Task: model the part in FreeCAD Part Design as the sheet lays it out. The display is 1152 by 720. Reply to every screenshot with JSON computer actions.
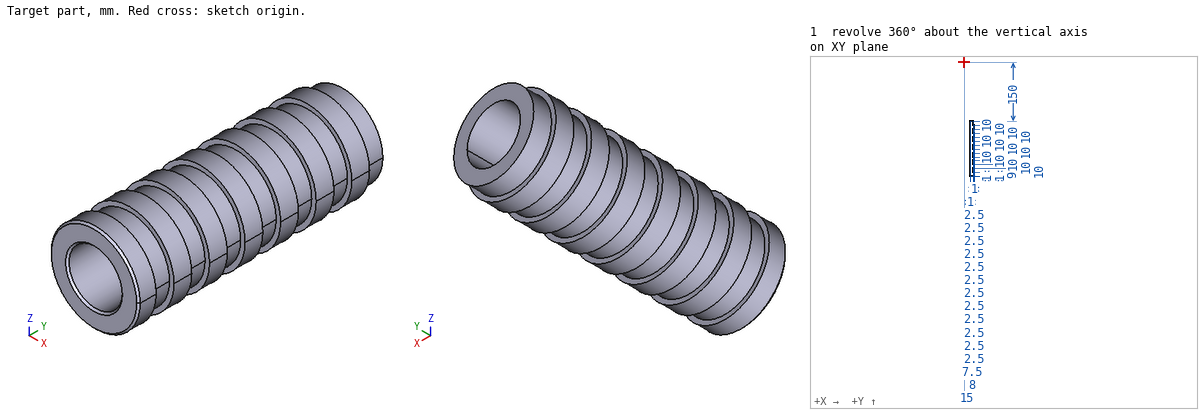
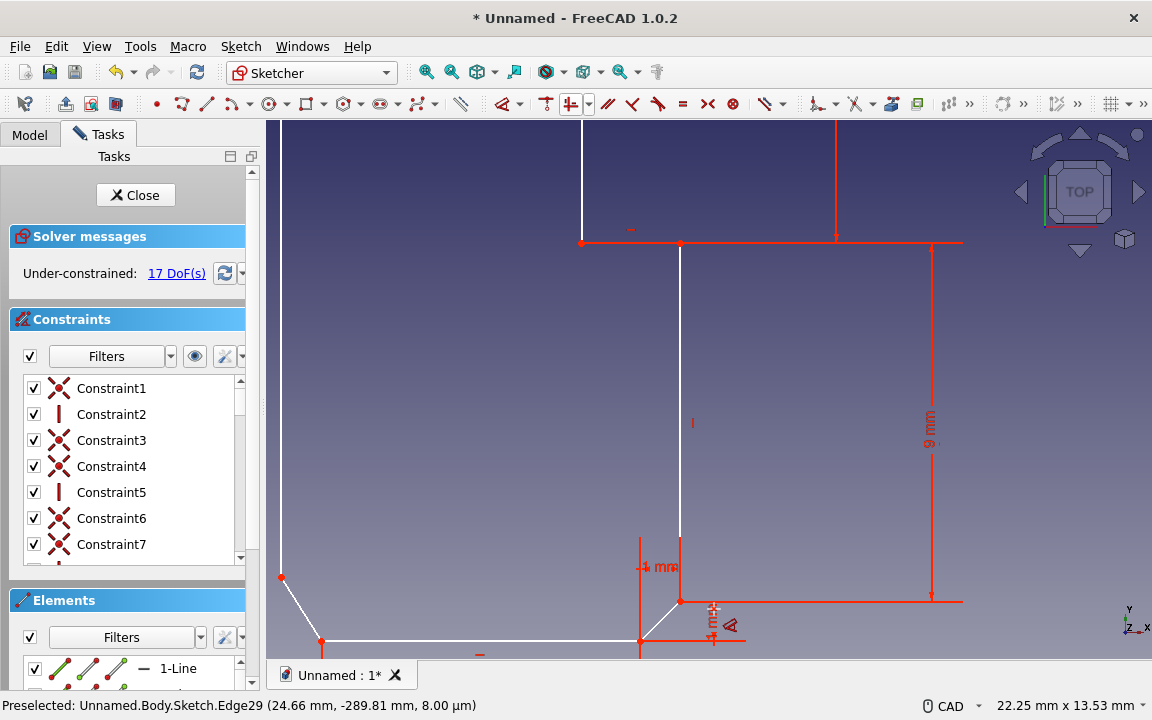
{"action": "left_click", "coordinate": [310, 622]}
{"action": "left_click", "coordinate": [308, 544]}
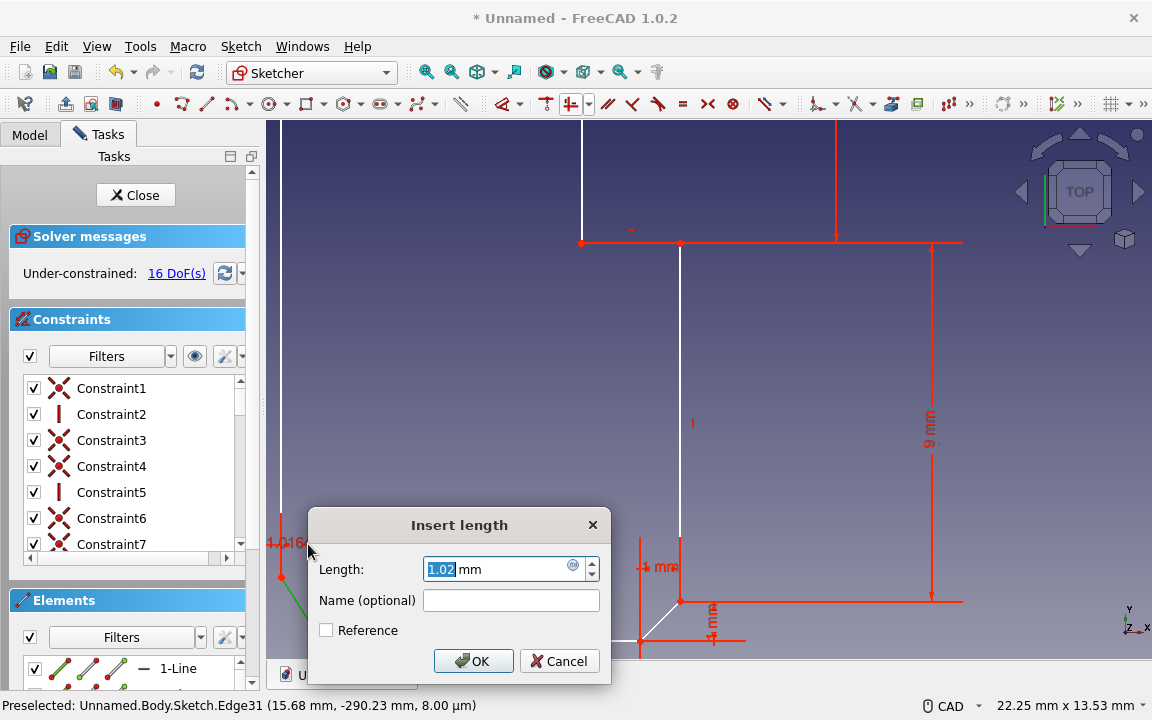
{"action": "type", "text": "1"}
{"action": "key", "text": "Return"}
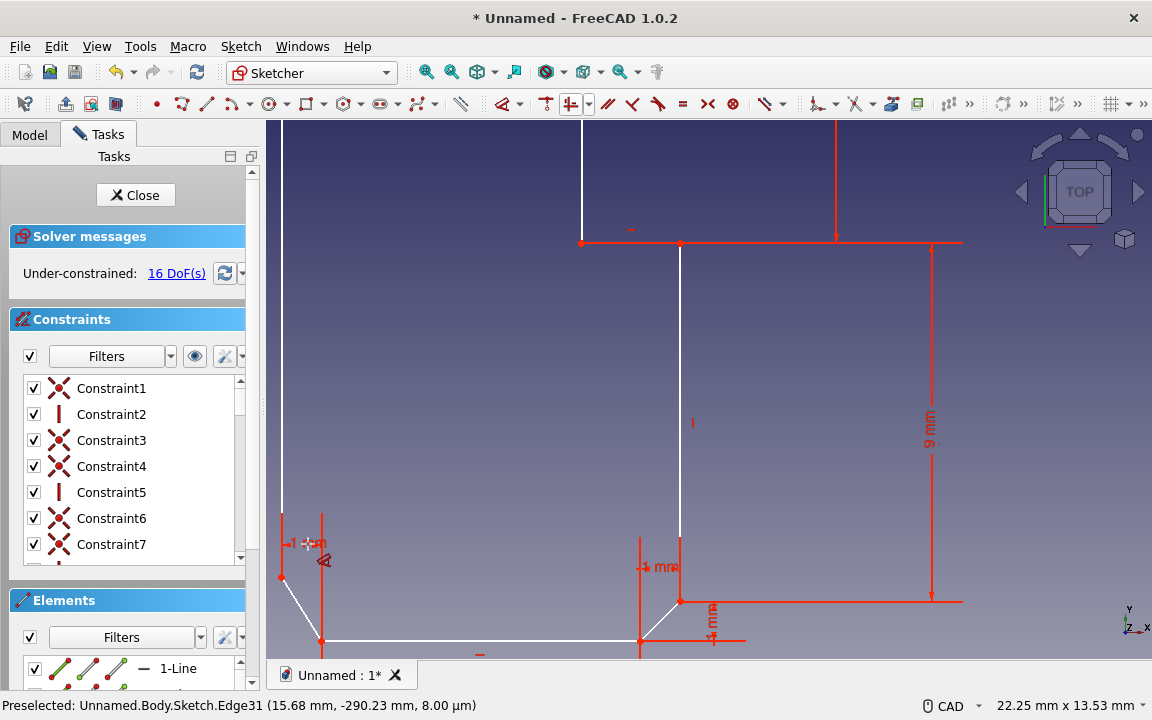
{"action": "left_click", "coordinate": [310, 622]}
{"action": "left_click", "coordinate": [356, 604]}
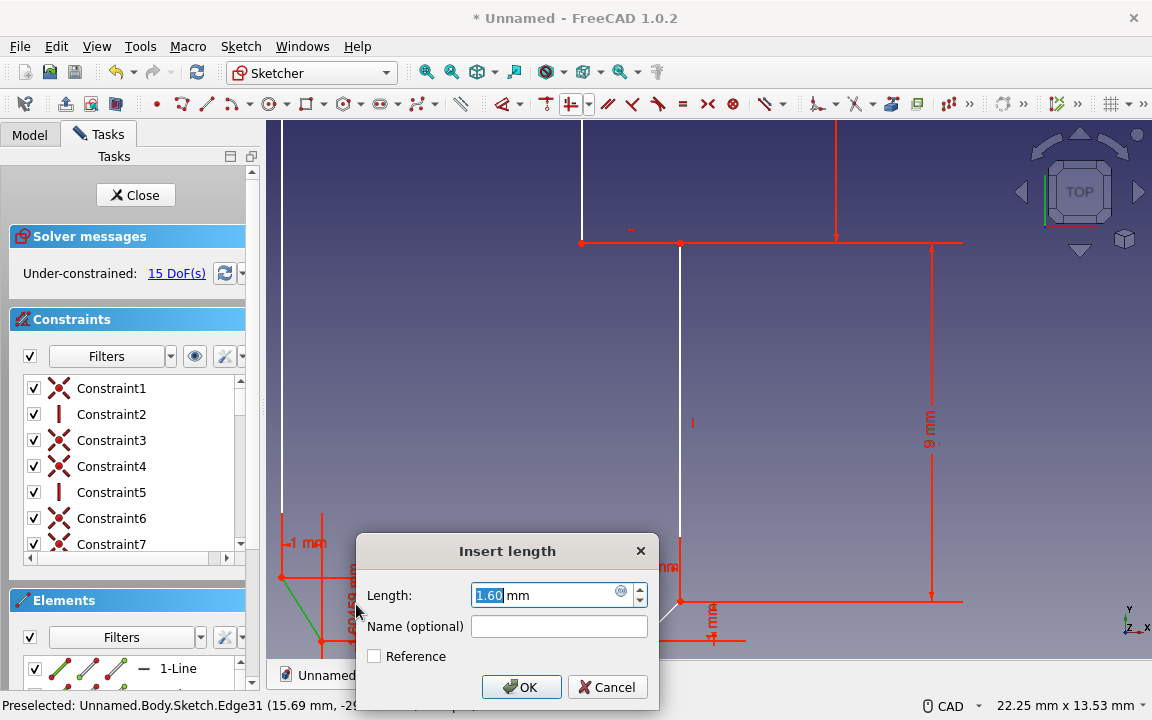
{"action": "type", "text": "1"}
{"action": "key", "text": "Return"}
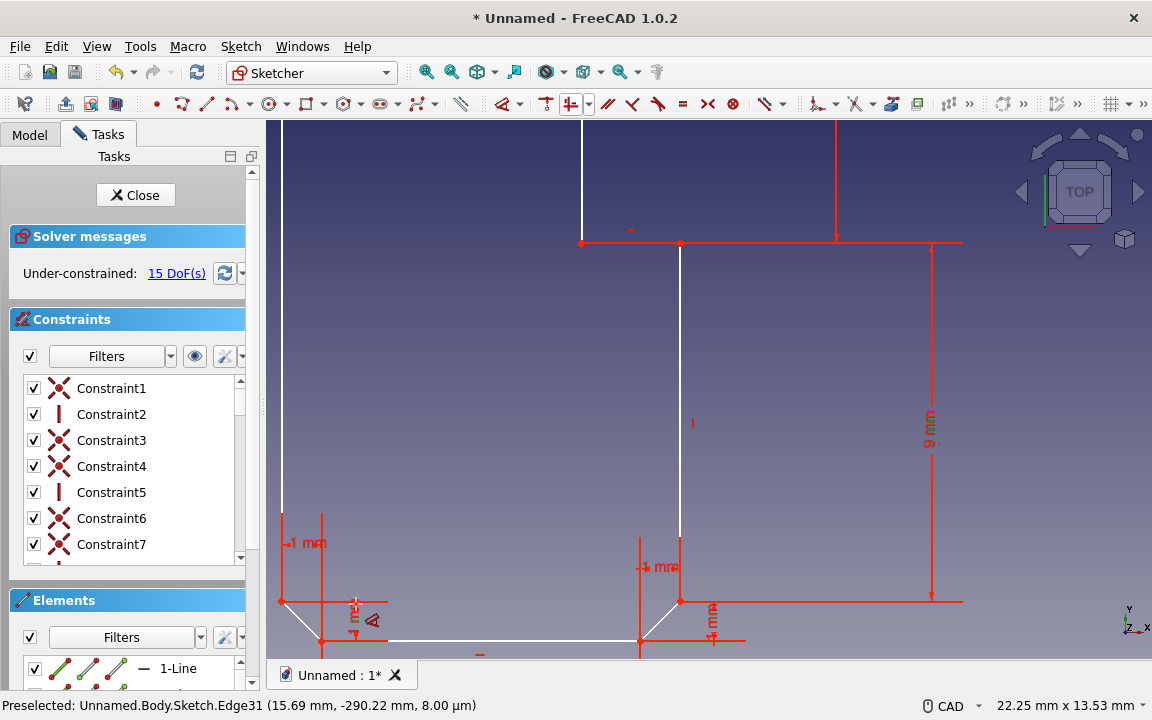
{"action": "scroll", "coordinate": [656, 581], "scroll_direction": "down", "scroll_amount": 17}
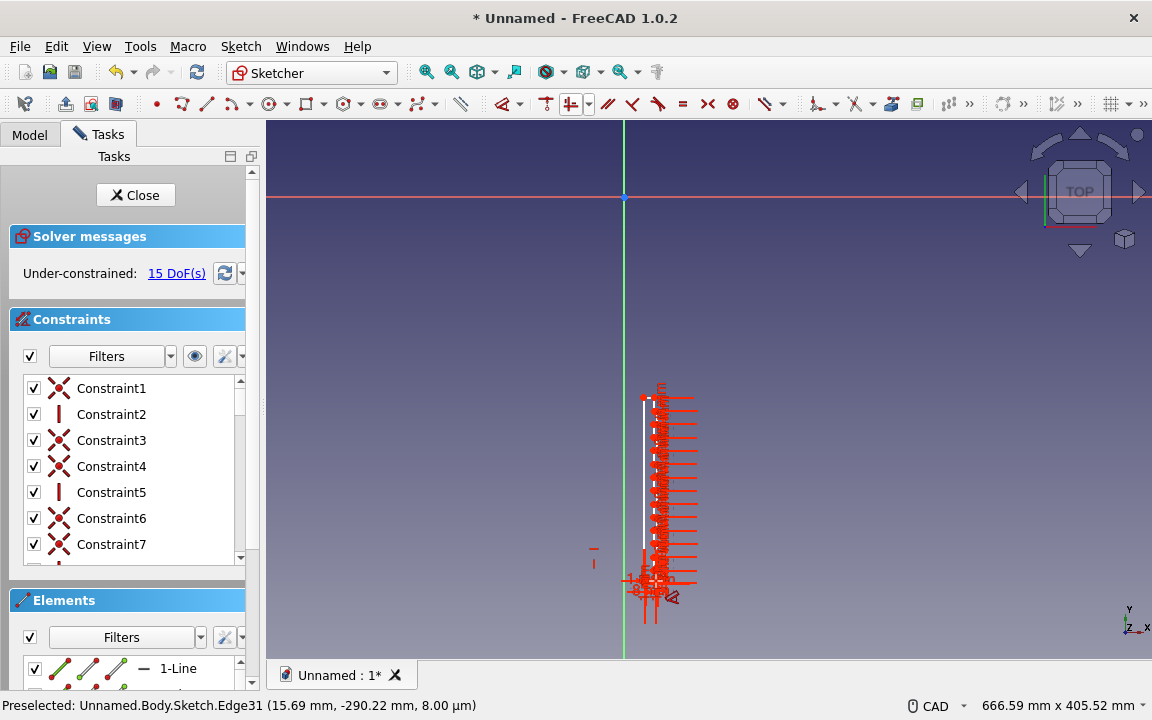
{"action": "scroll", "coordinate": [647, 398], "scroll_direction": "up", "scroll_amount": 8}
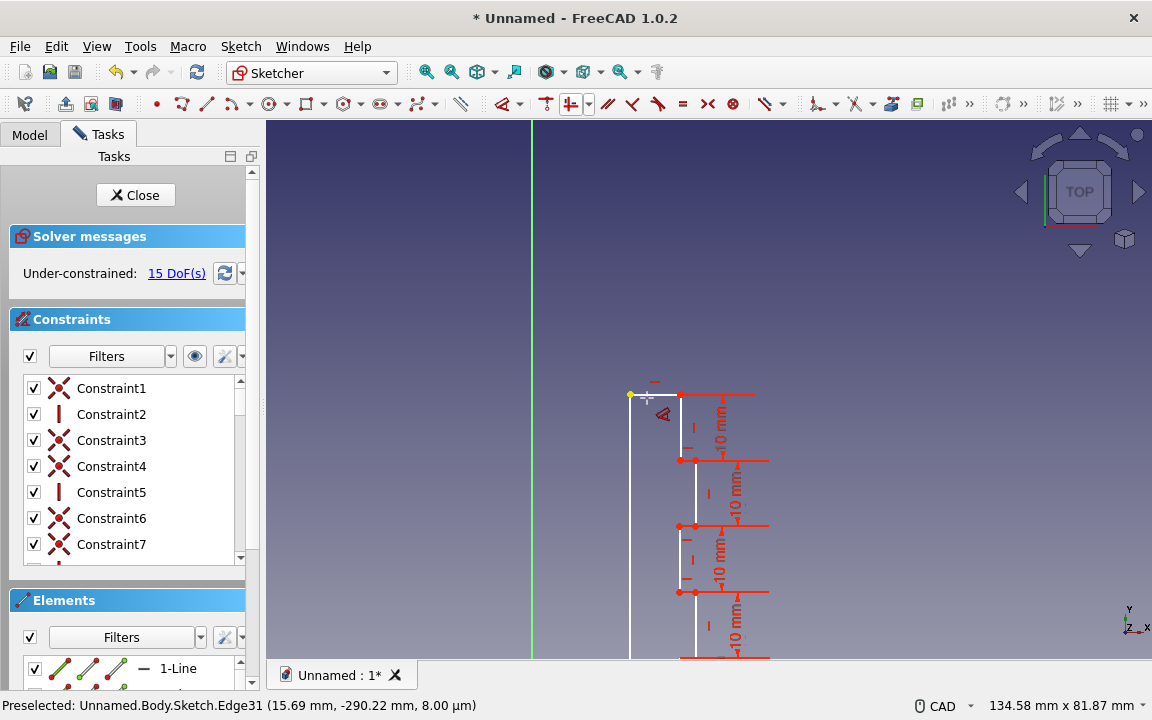
{"action": "left_click", "coordinate": [645, 395]}
{"action": "left_click", "coordinate": [644, 429]}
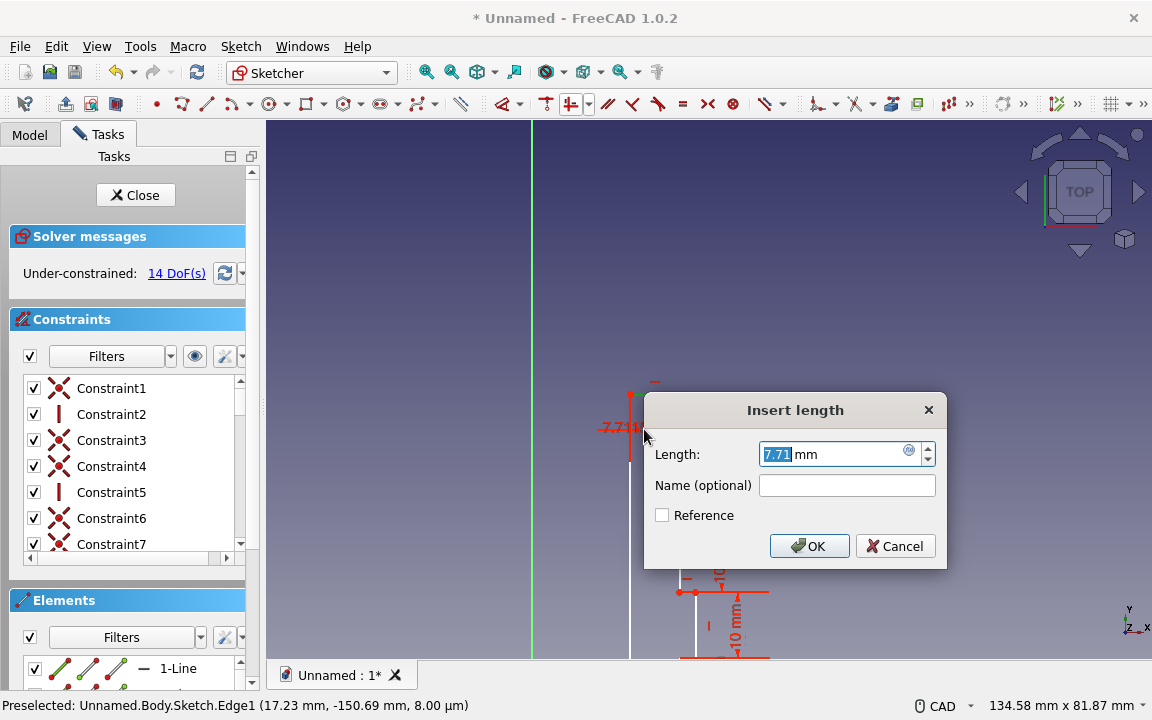
{"action": "type", "text": "7.5"}
{"action": "key", "text": "Return"}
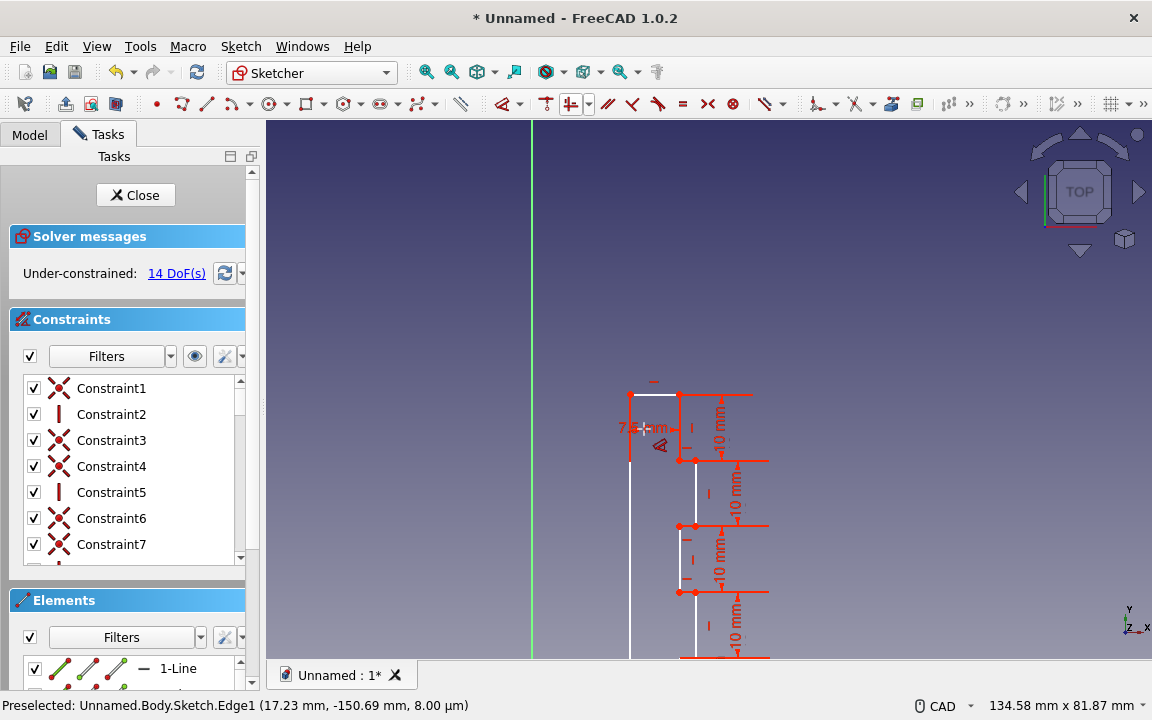
{"action": "scroll", "coordinate": [688, 461], "scroll_direction": "up", "scroll_amount": 5}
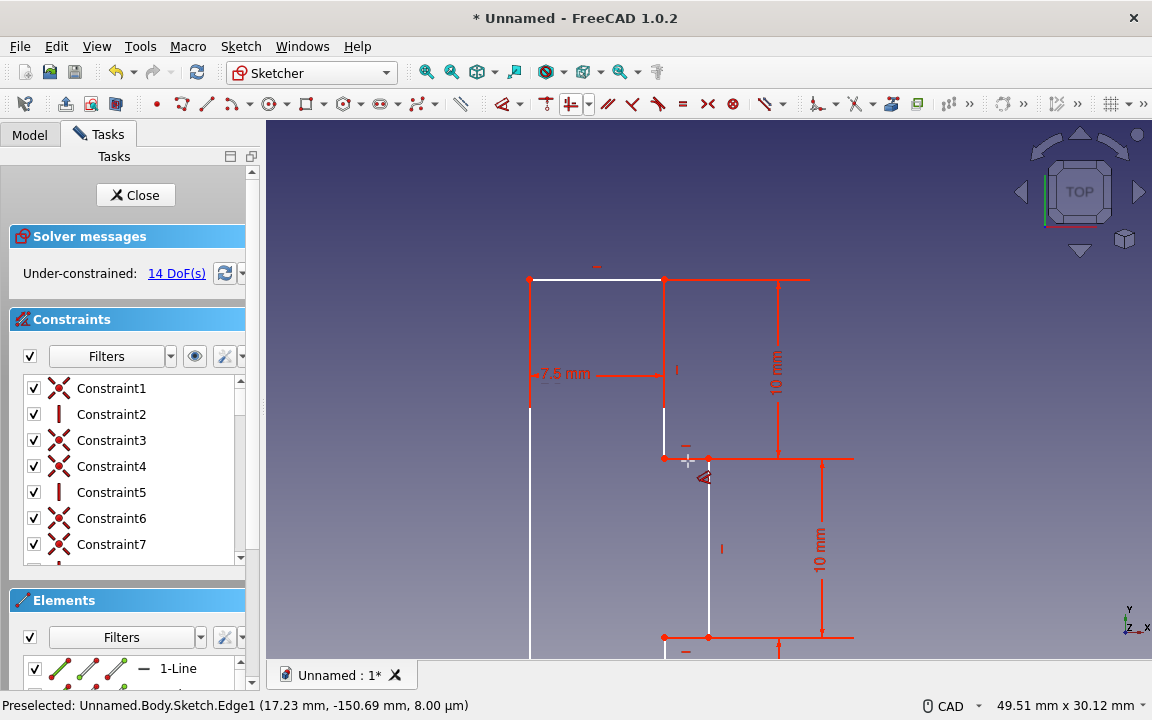
{"action": "left_click", "coordinate": [686, 459]}
{"action": "left_click", "coordinate": [686, 493]}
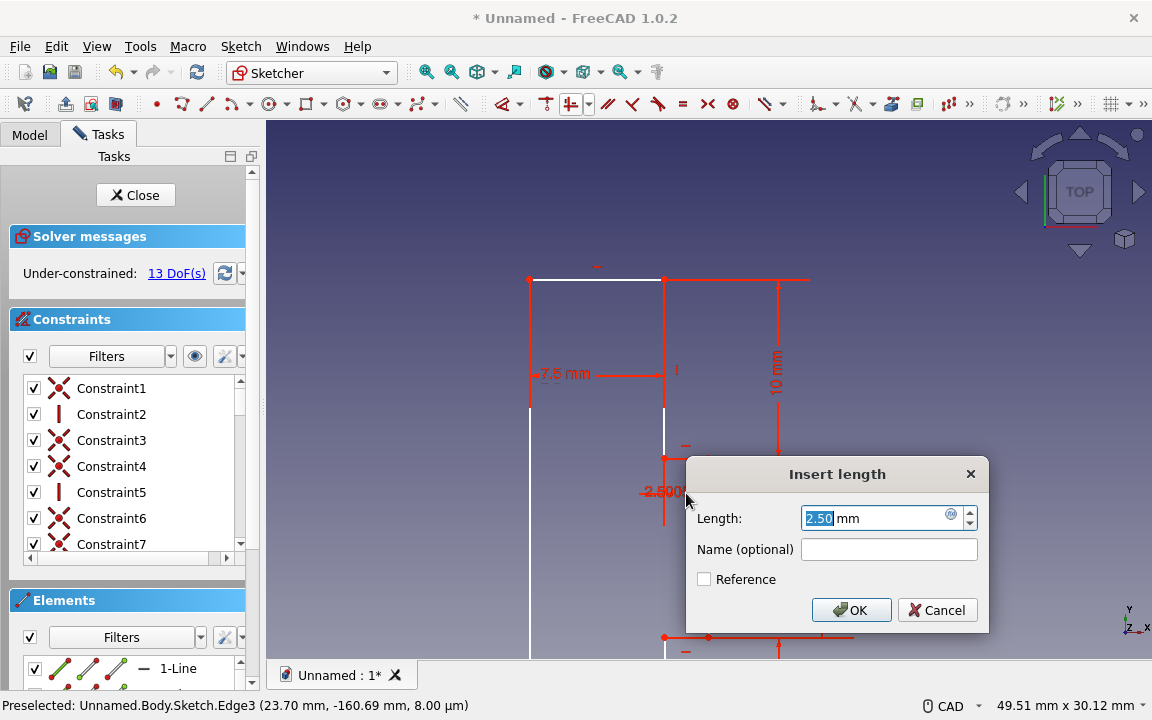
{"action": "type", "text": "2.5"}
{"action": "key", "text": "Return"}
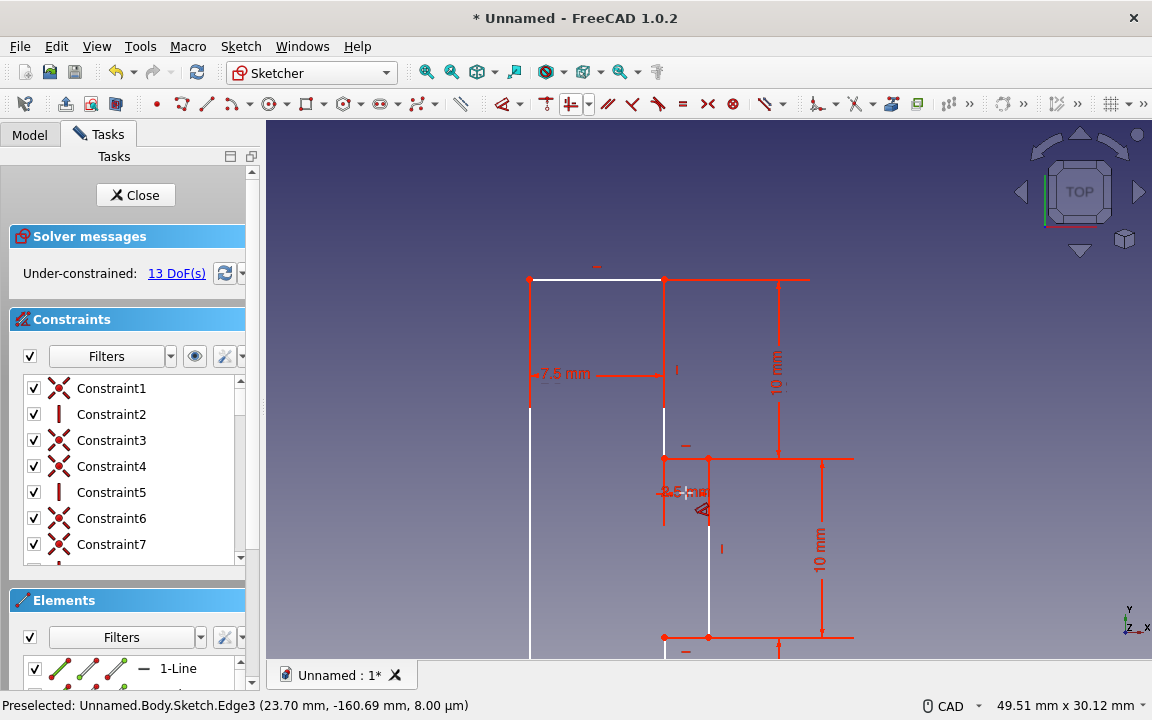
{"action": "scroll", "coordinate": [651, 403], "scroll_direction": "down", "scroll_amount": 14}